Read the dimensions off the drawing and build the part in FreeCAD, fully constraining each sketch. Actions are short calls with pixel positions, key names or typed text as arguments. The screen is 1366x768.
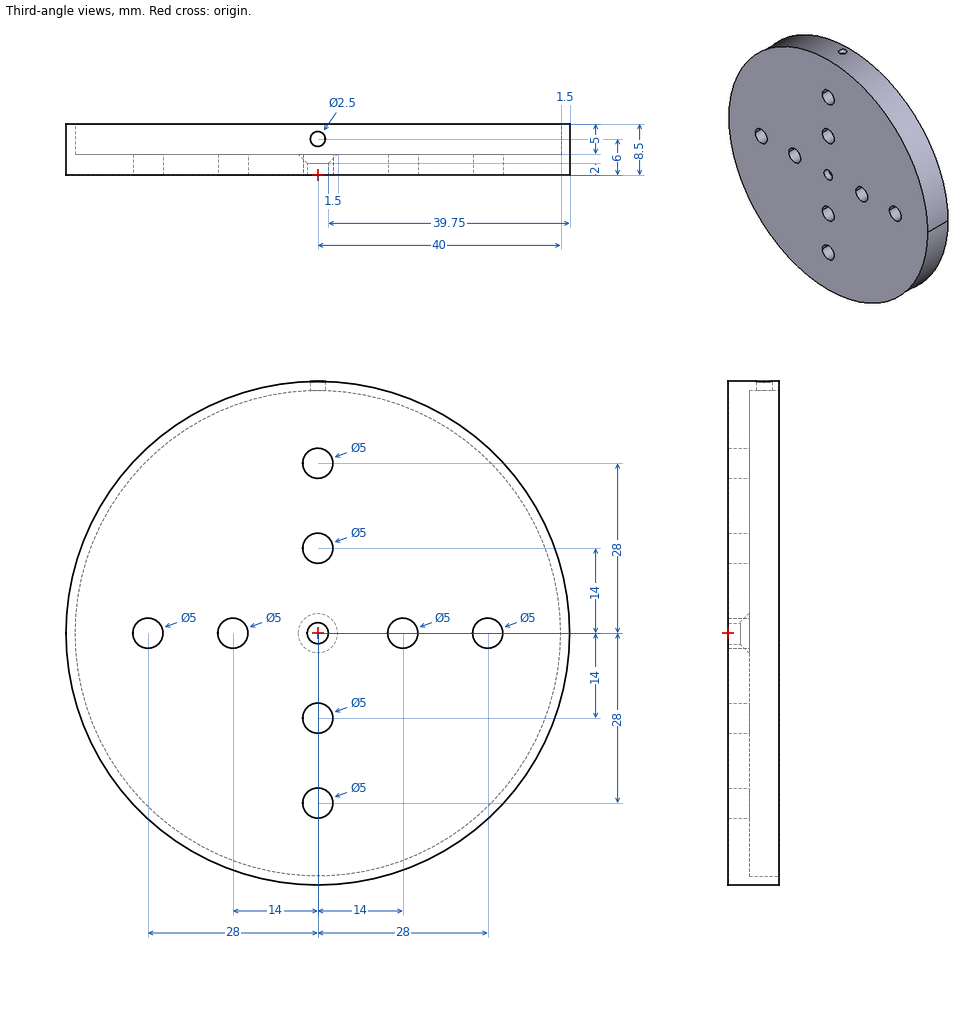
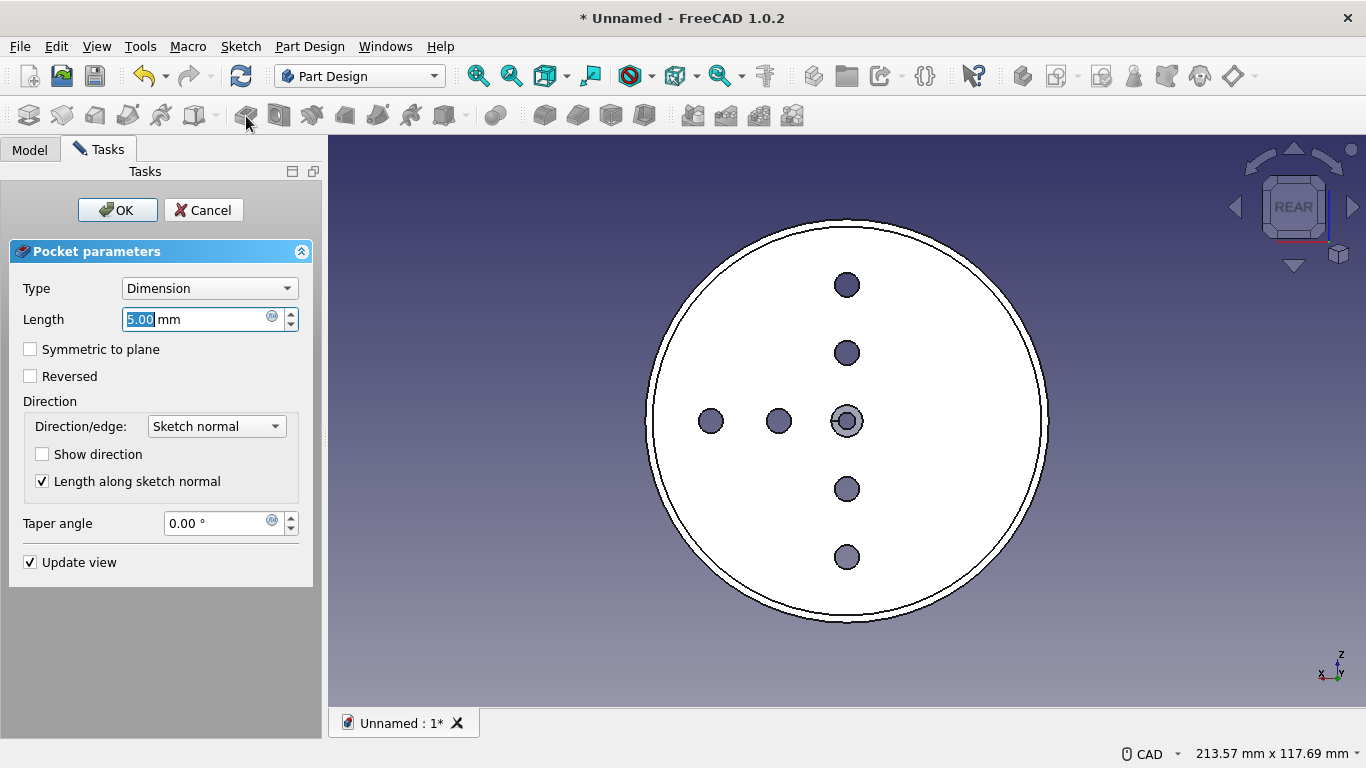
click(210, 288)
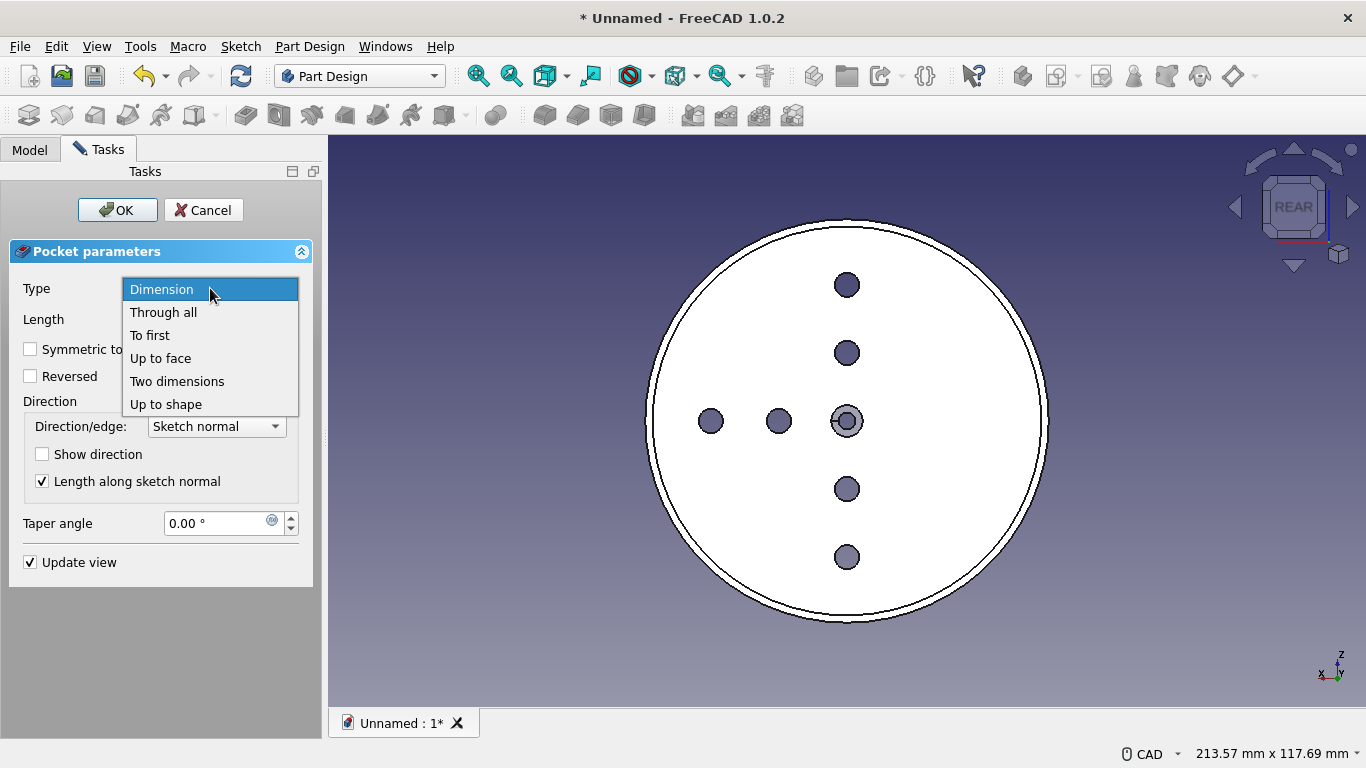
click(208, 336)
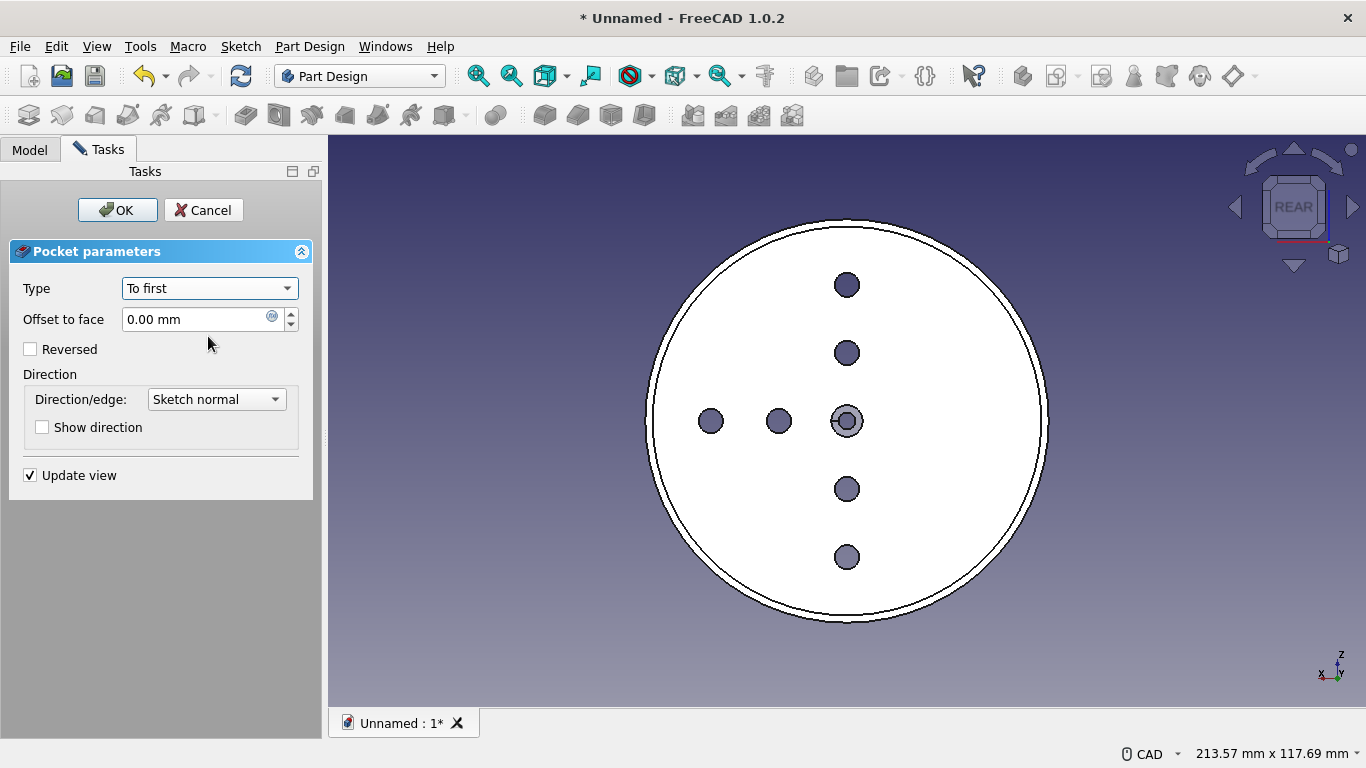
click(118, 210)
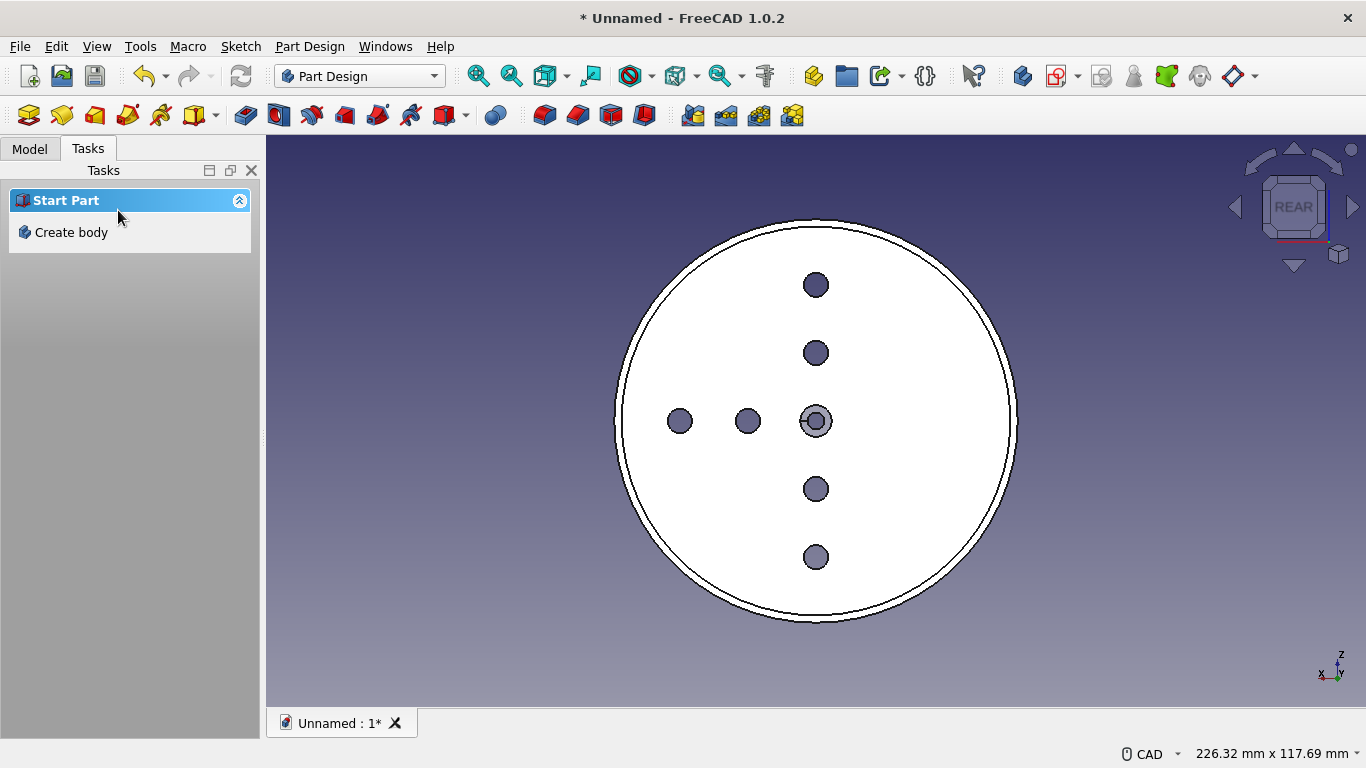
click(927, 420)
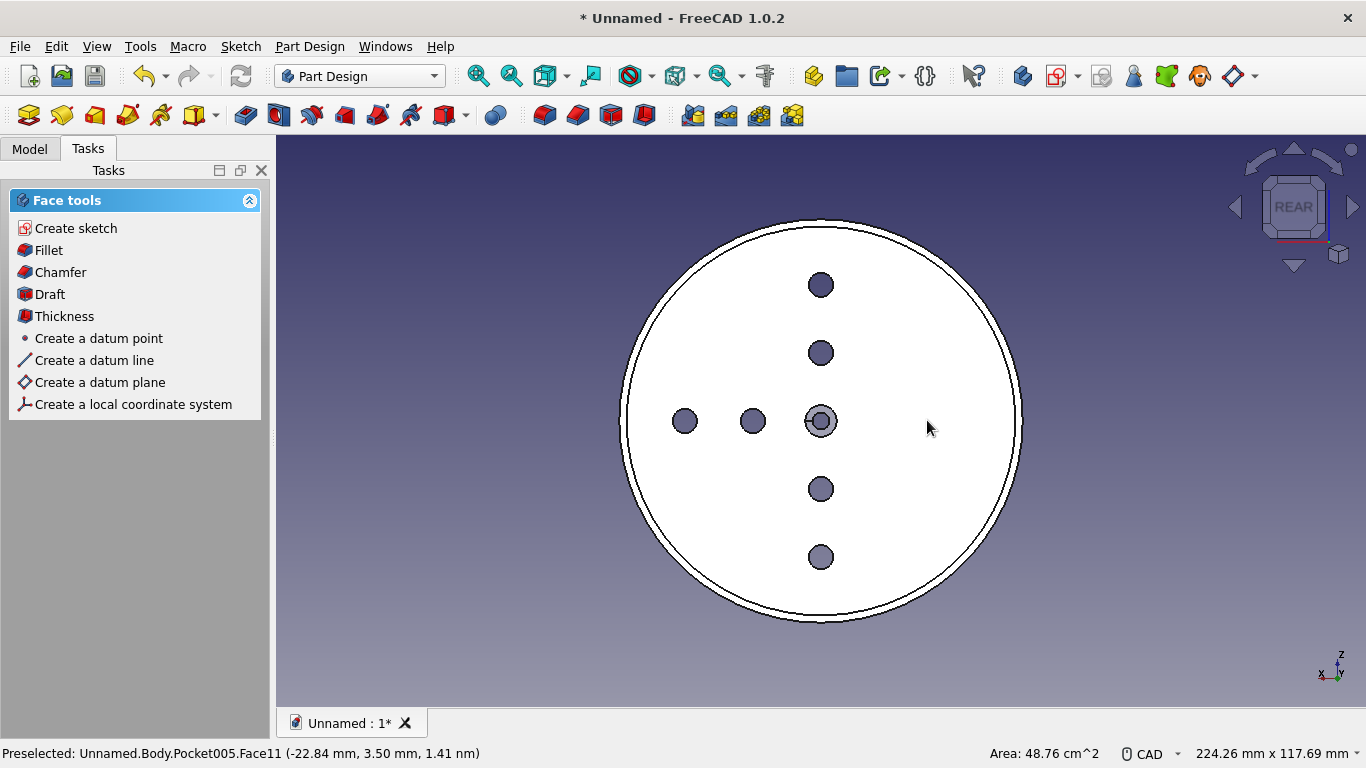
click(1056, 76)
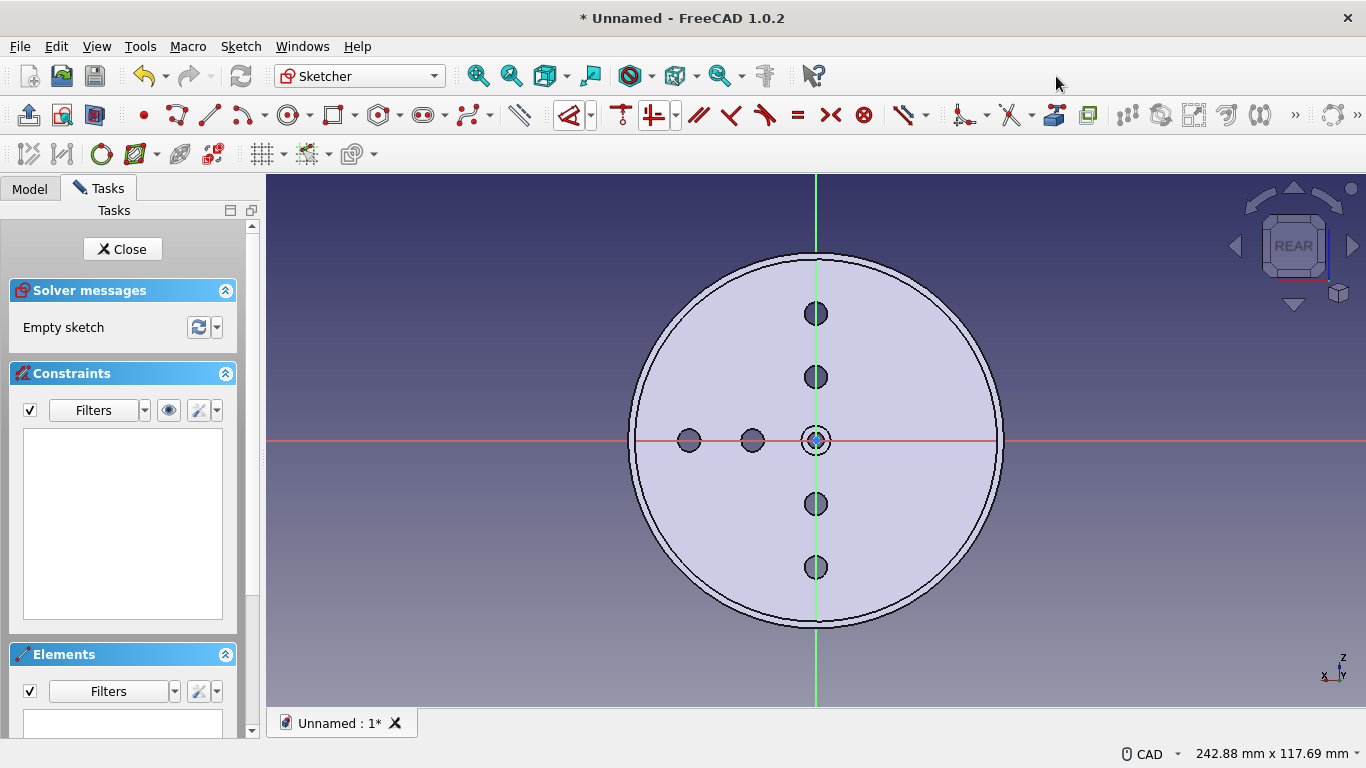
scroll(890, 441, up, 13)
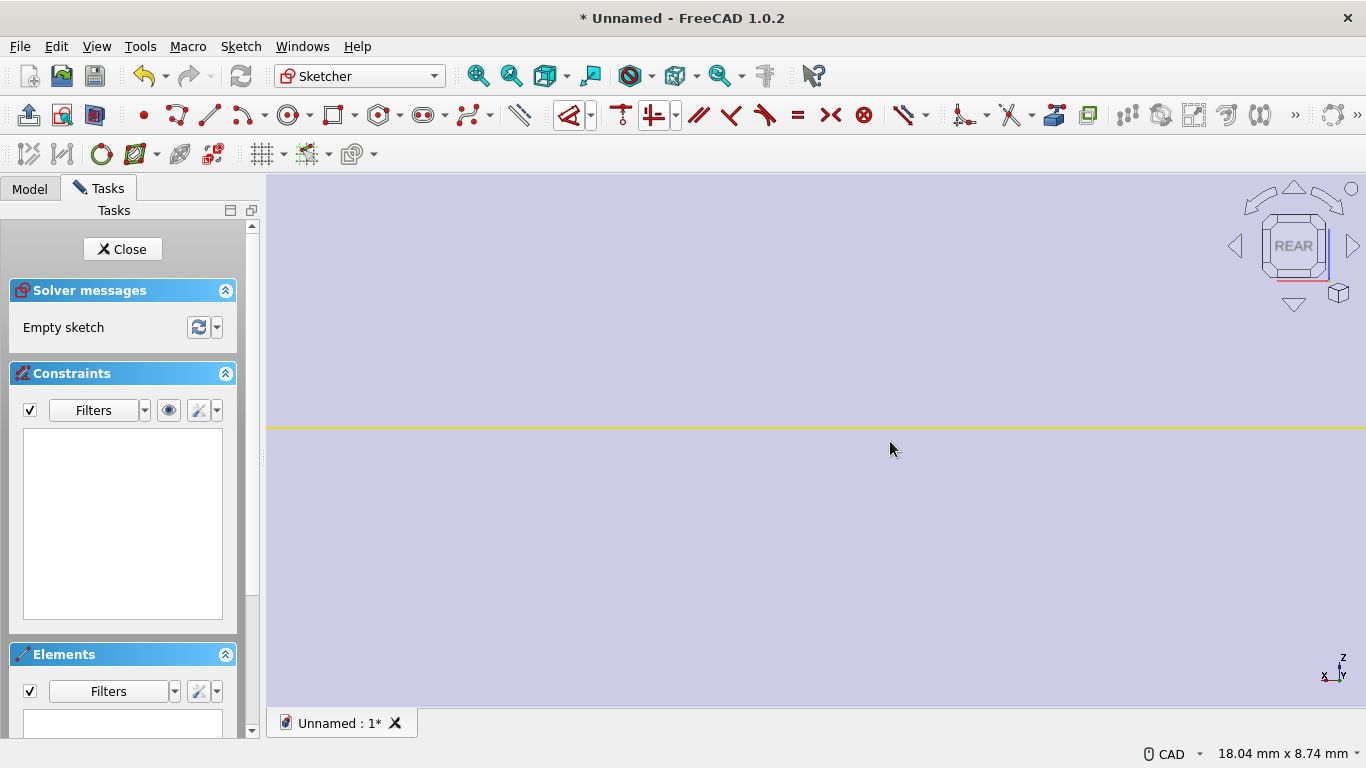
click(288, 116)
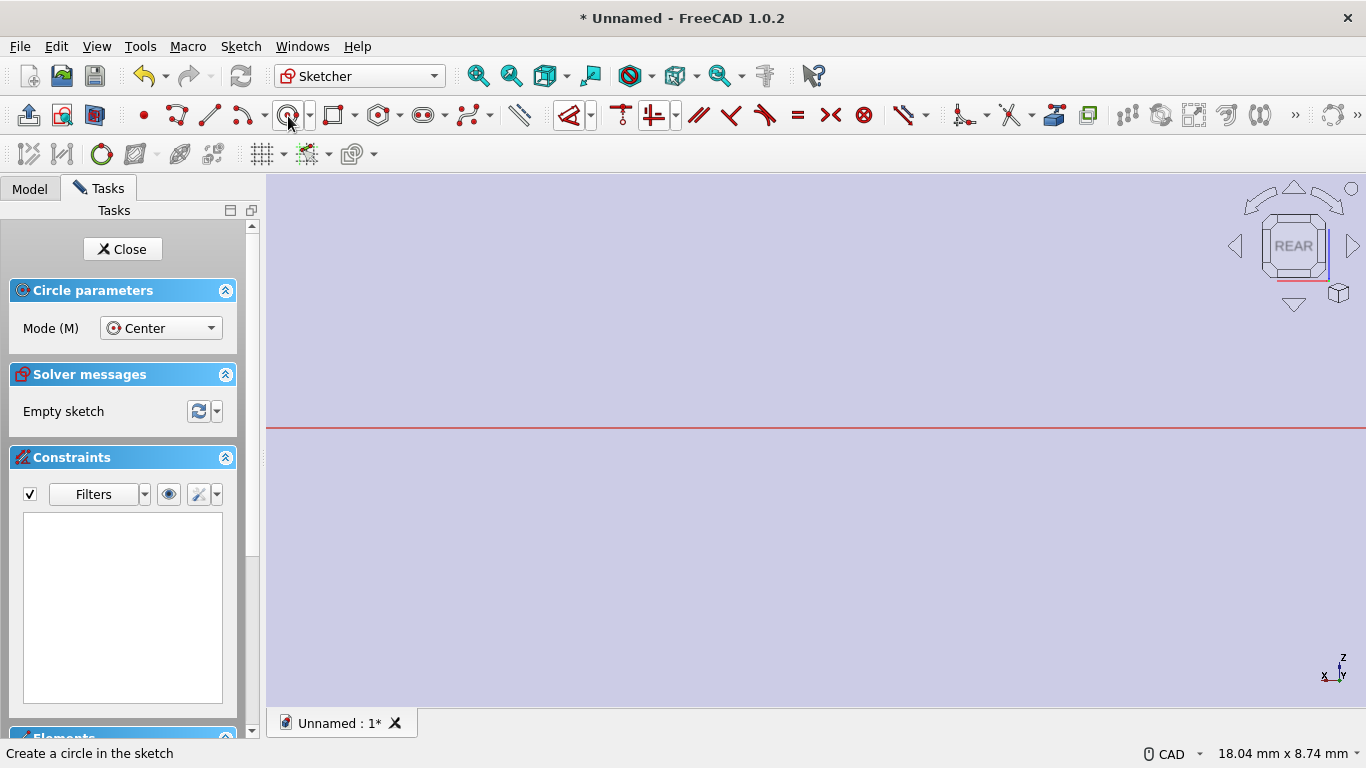
click(740, 428)
click(848, 320)
key(Escape)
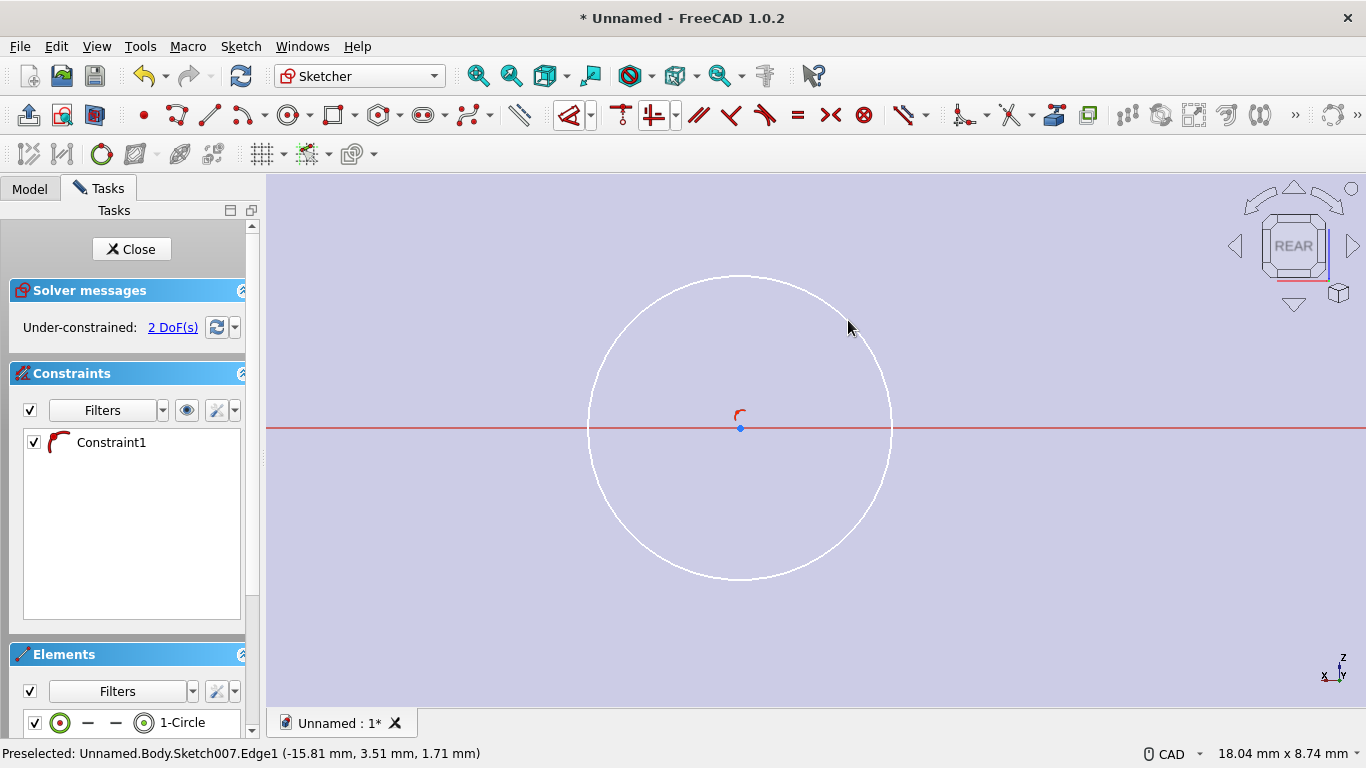
click(847, 320)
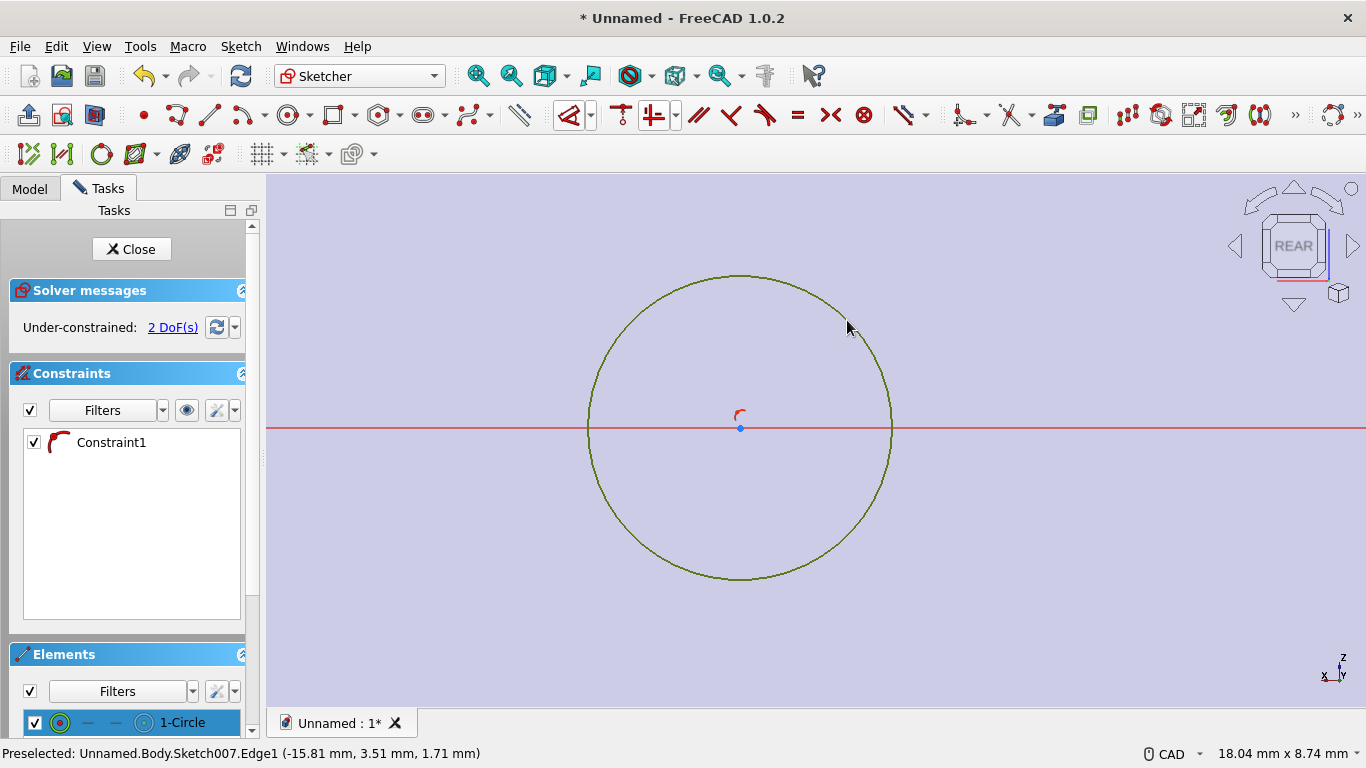
click(590, 116)